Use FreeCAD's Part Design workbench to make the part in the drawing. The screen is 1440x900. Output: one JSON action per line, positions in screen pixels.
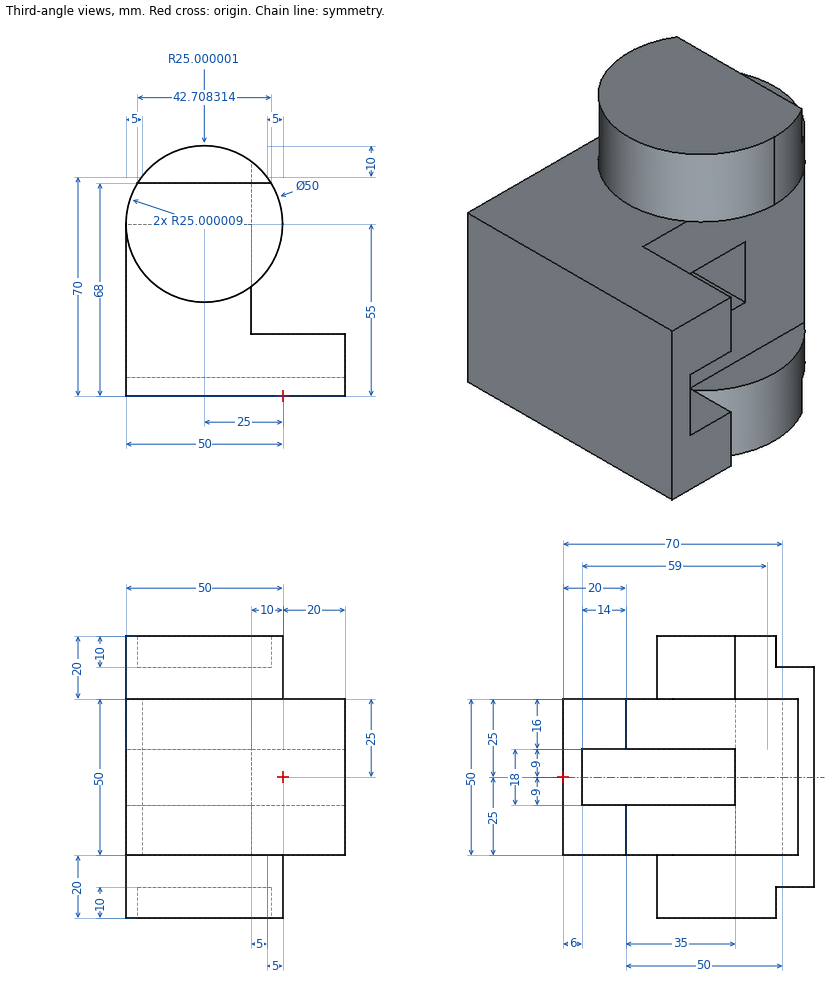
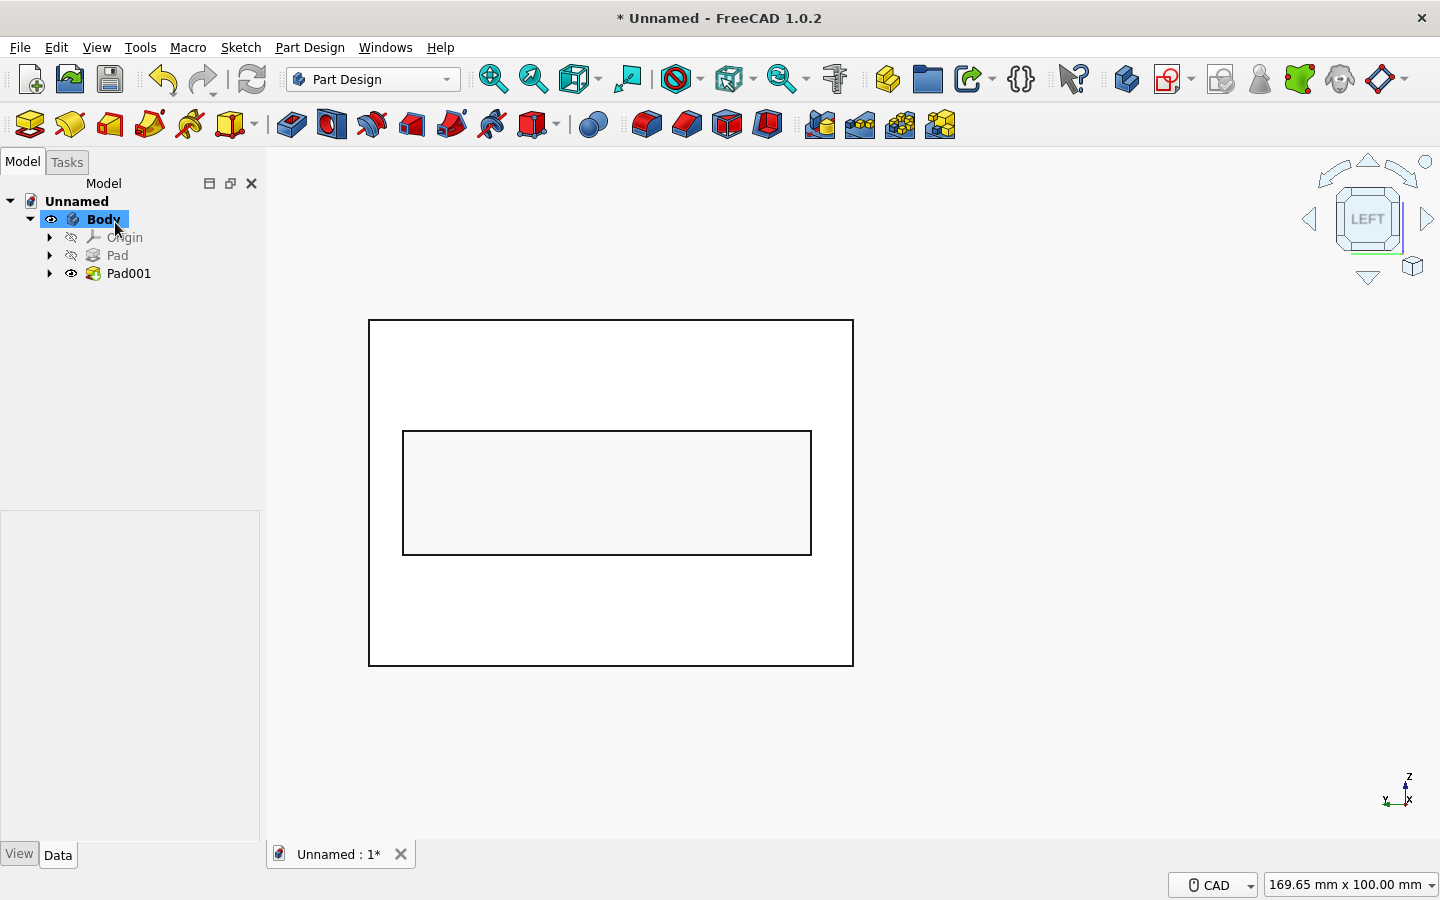
{"action": "key", "text": "0"}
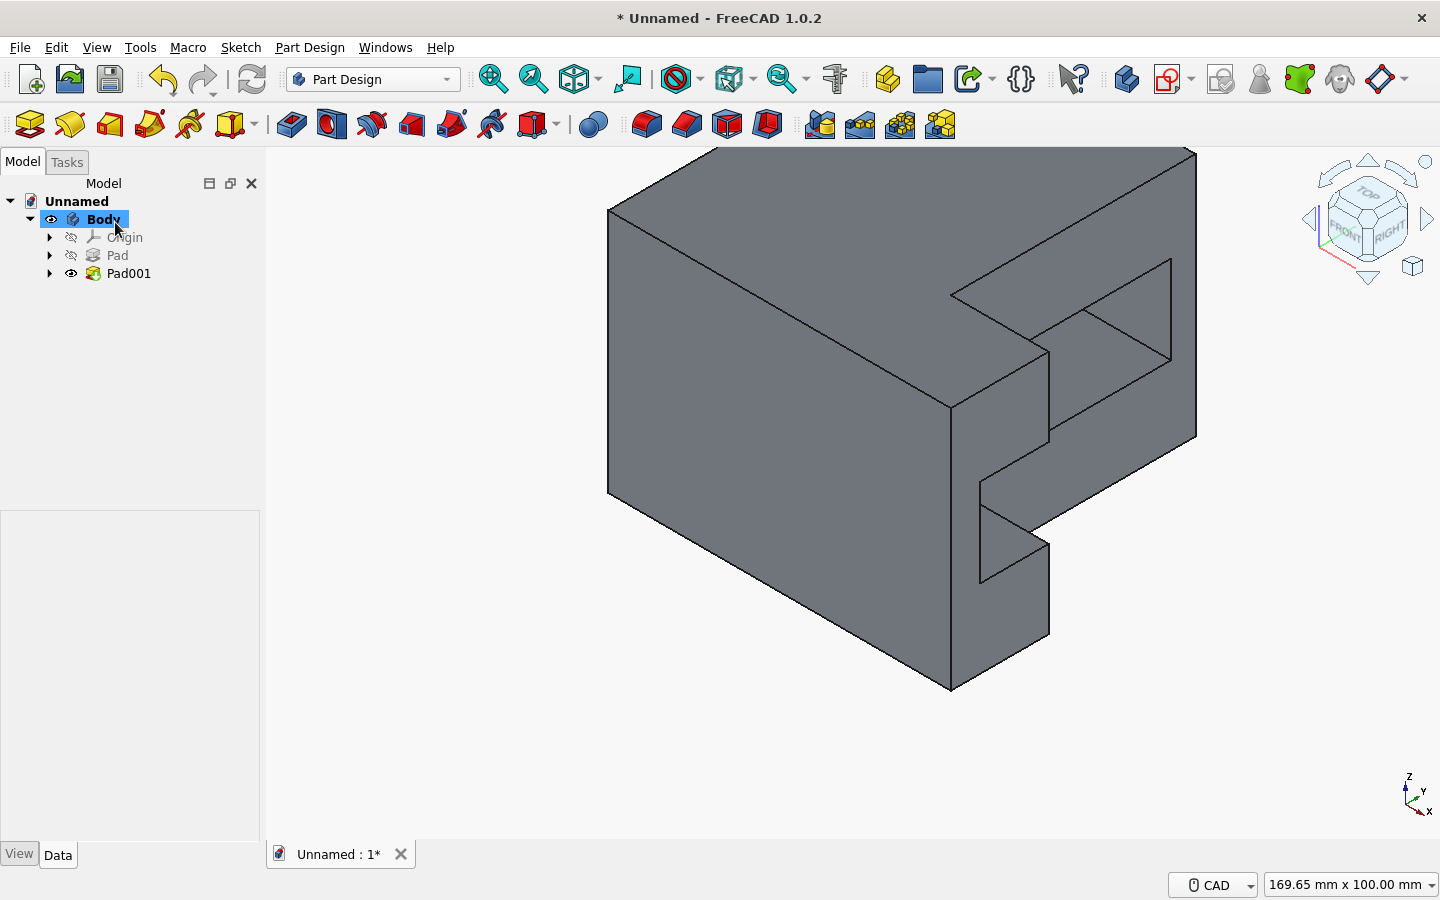
{"action": "left_click", "coordinate": [494, 80]}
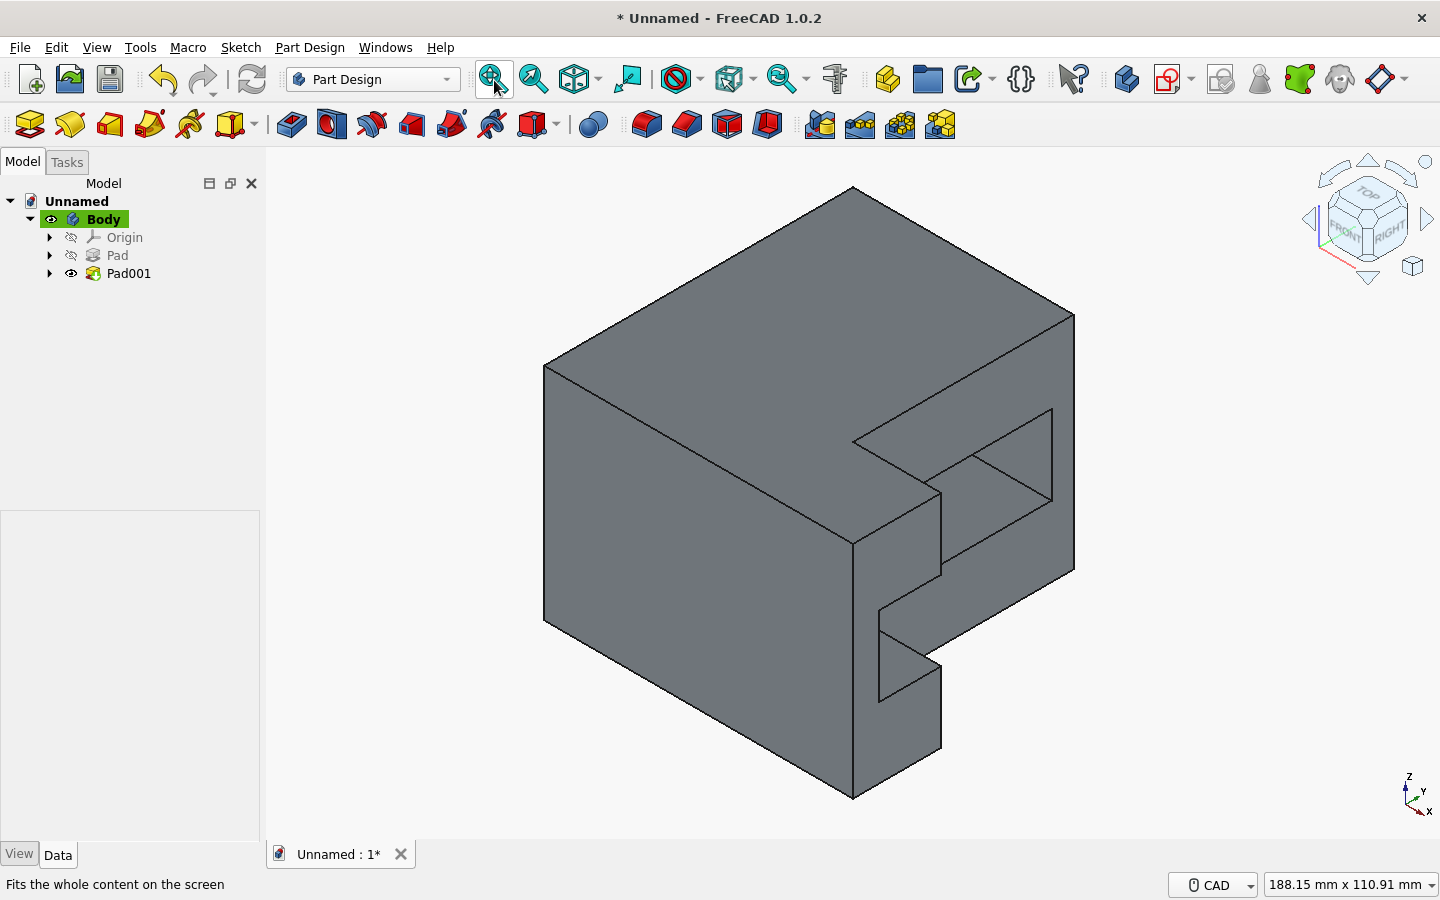
{"action": "left_click", "coordinate": [853, 314]}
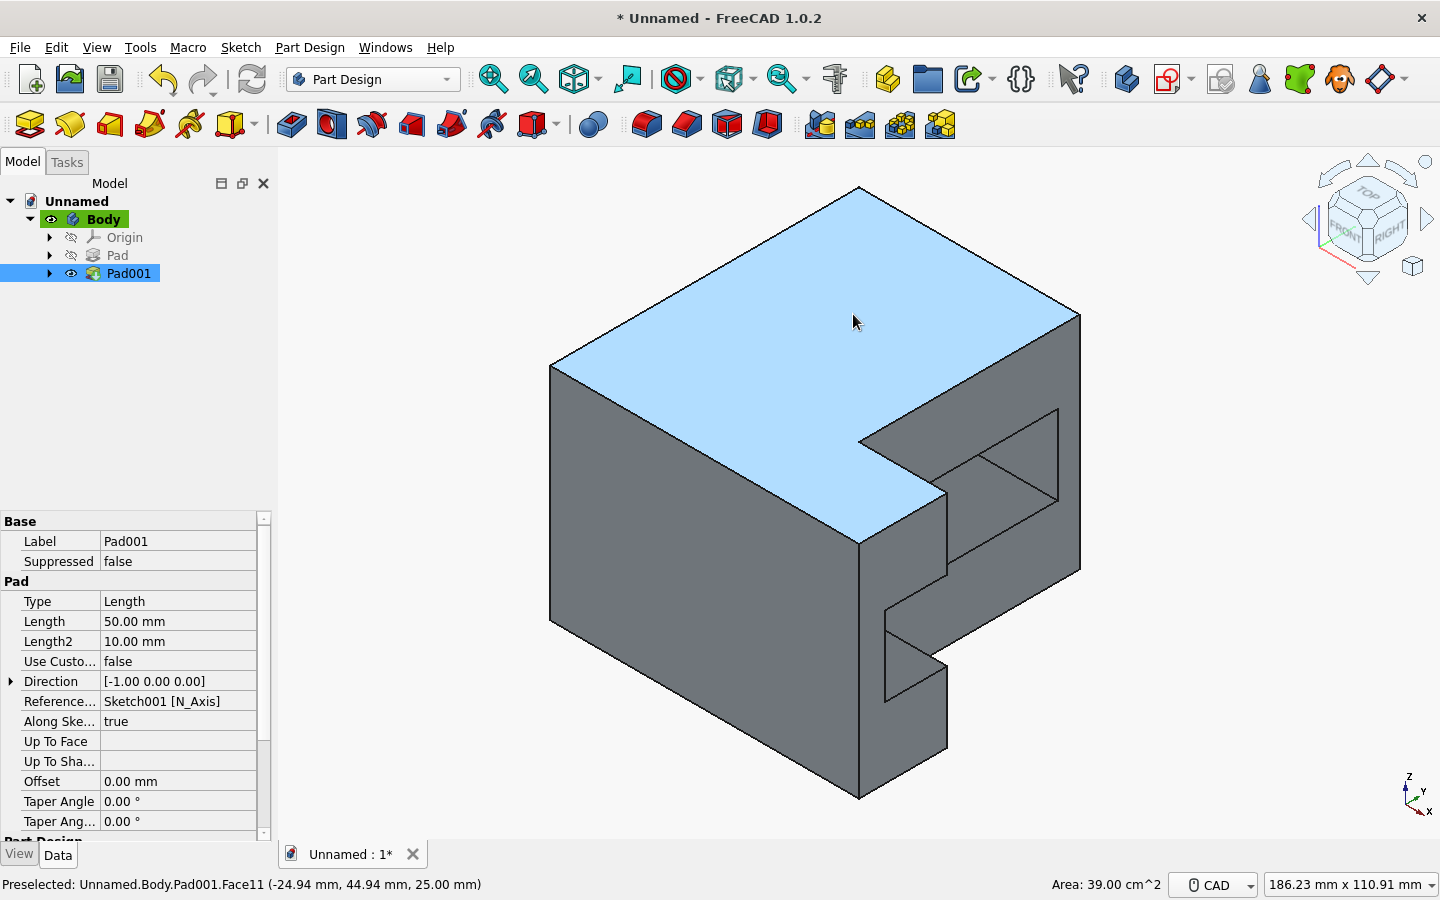
{"action": "left_click", "coordinate": [1168, 80]}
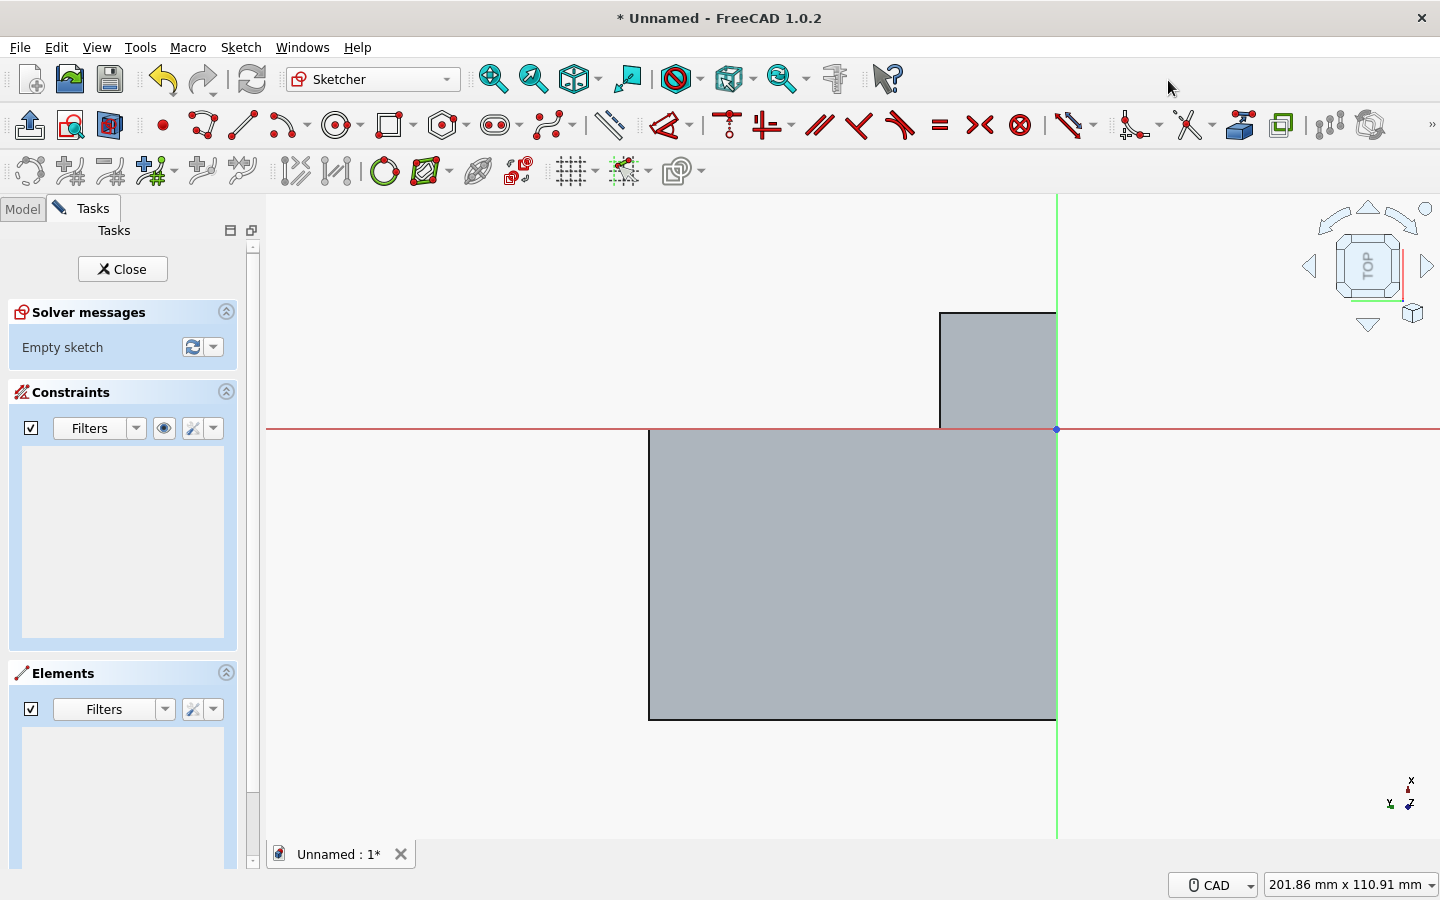
{"action": "scroll", "coordinate": [904, 693], "scroll_direction": "up", "scroll_amount": 2}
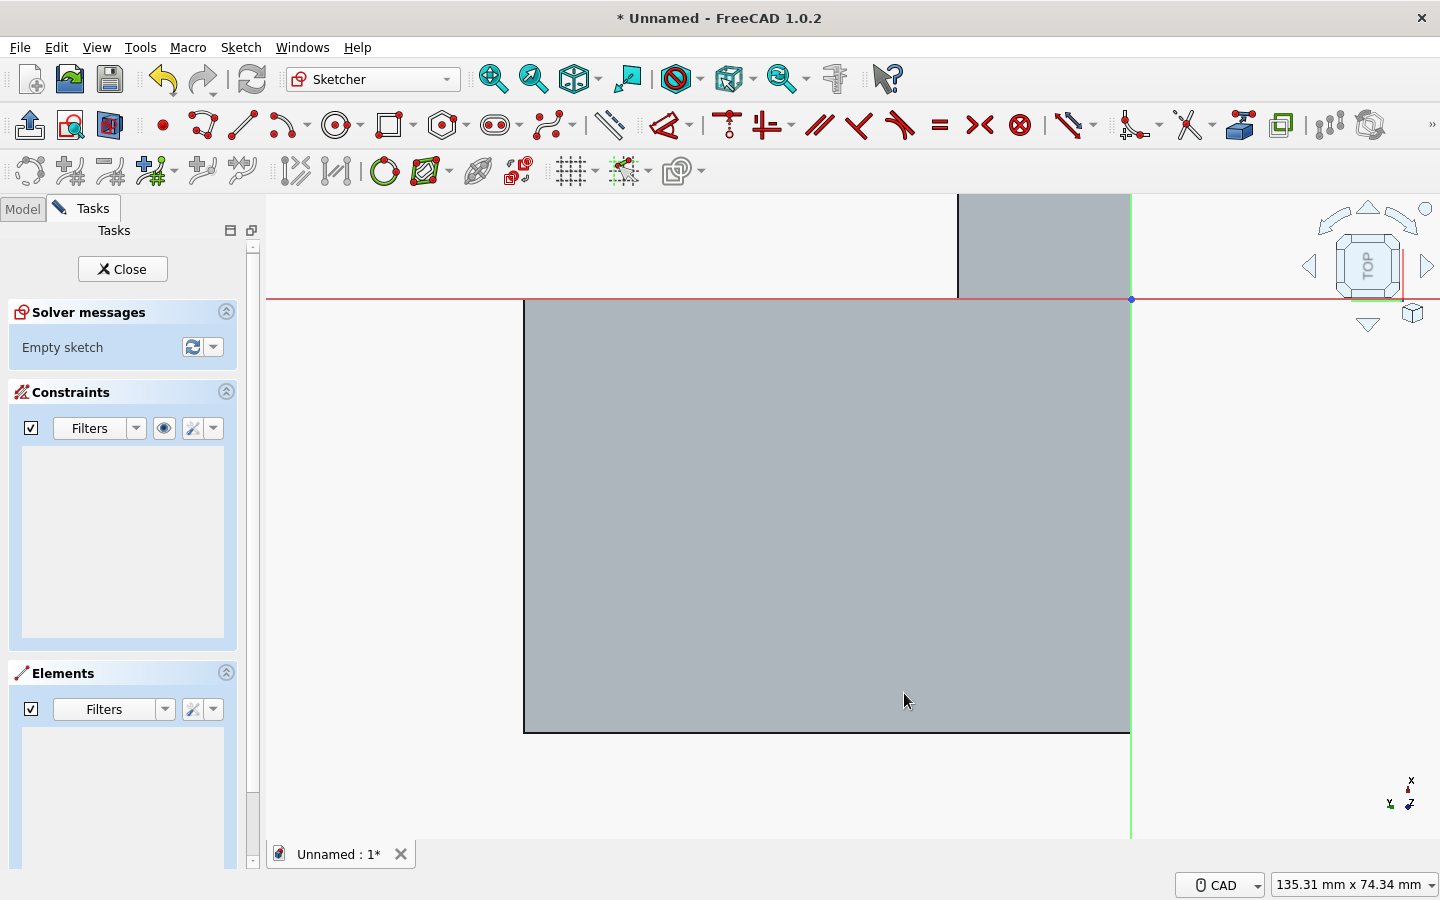
{"action": "left_click", "coordinate": [336, 126]}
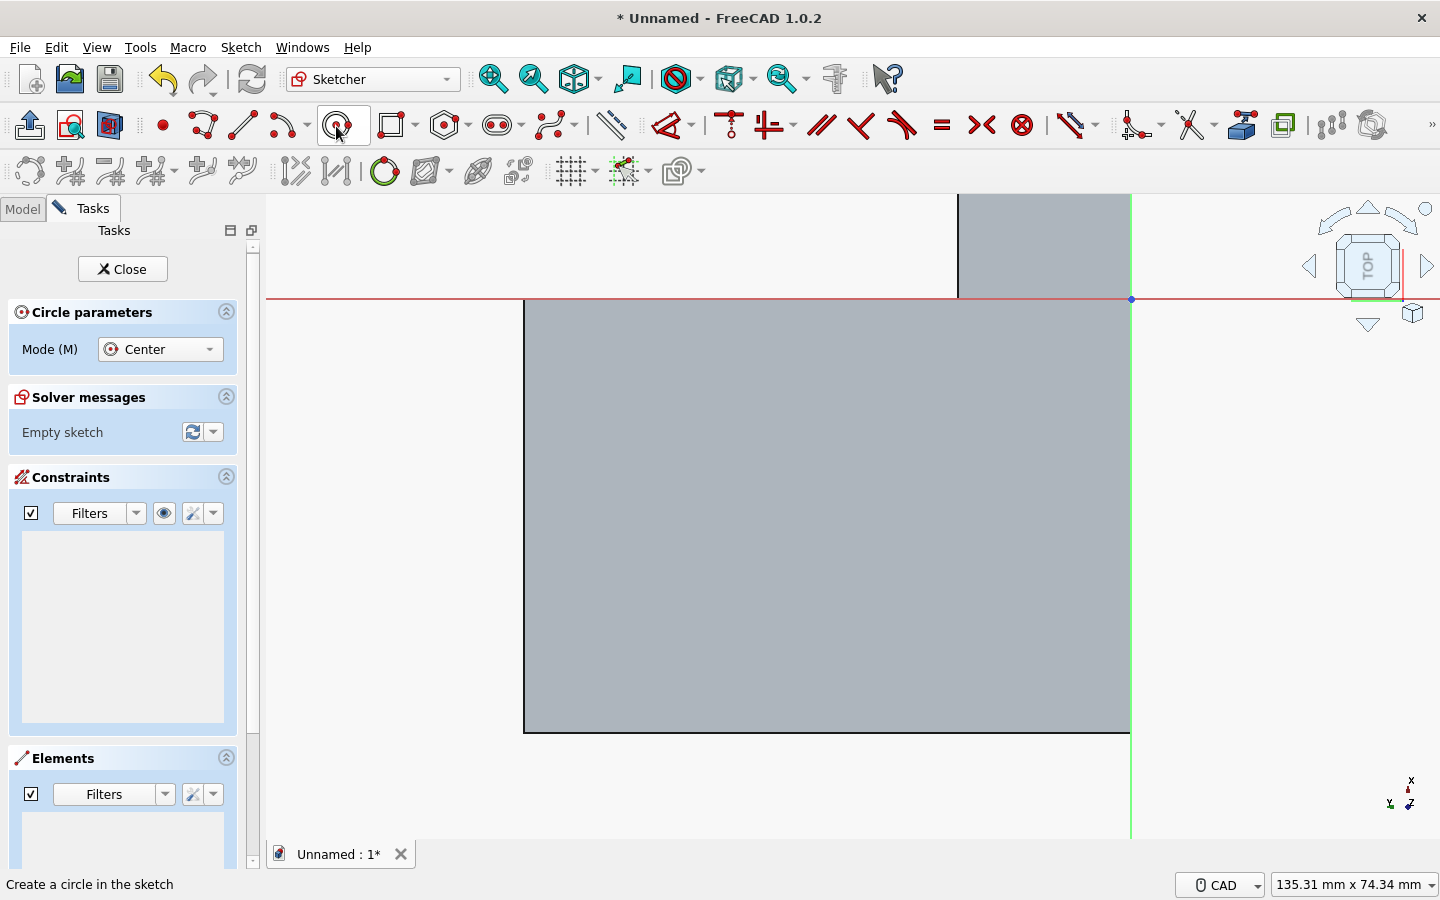
{"action": "left_click", "coordinate": [654, 516]}
{"action": "mouse_move", "coordinate": [808, 363]}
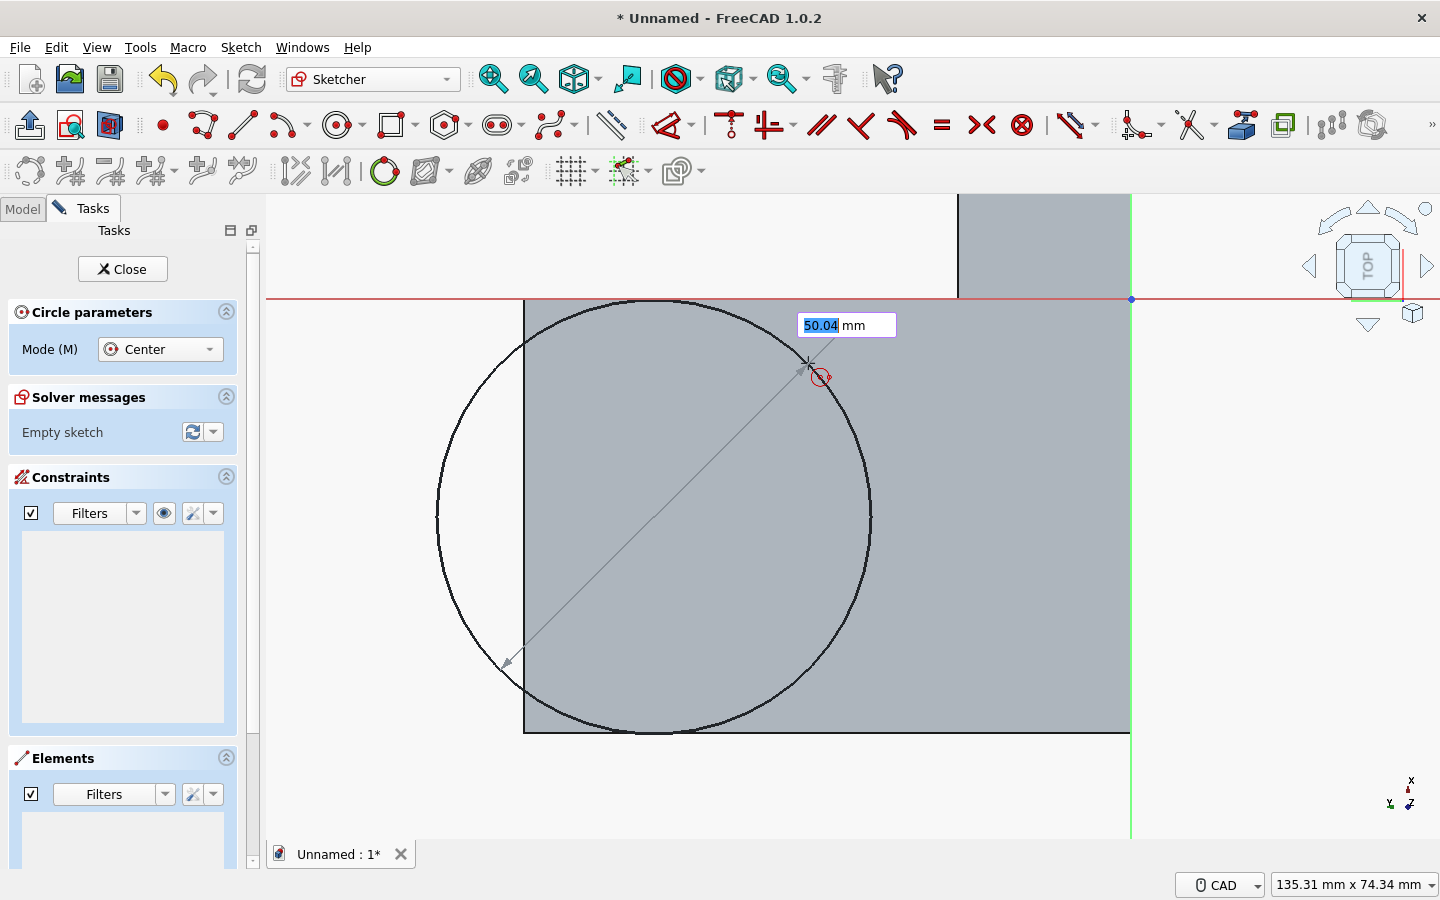
{"action": "type", "text": "50"}
{"action": "key", "text": "Return"}
{"action": "key", "text": "Escape"}